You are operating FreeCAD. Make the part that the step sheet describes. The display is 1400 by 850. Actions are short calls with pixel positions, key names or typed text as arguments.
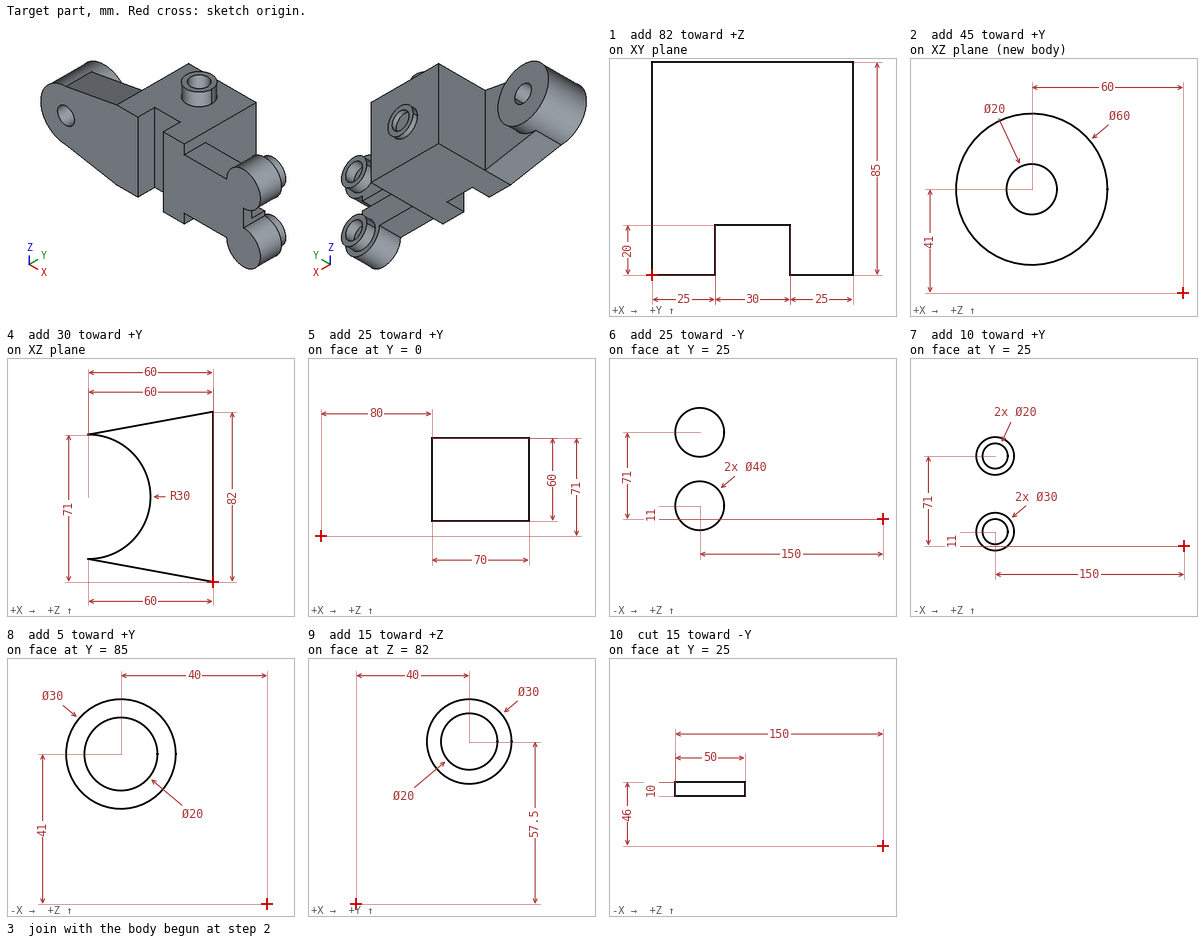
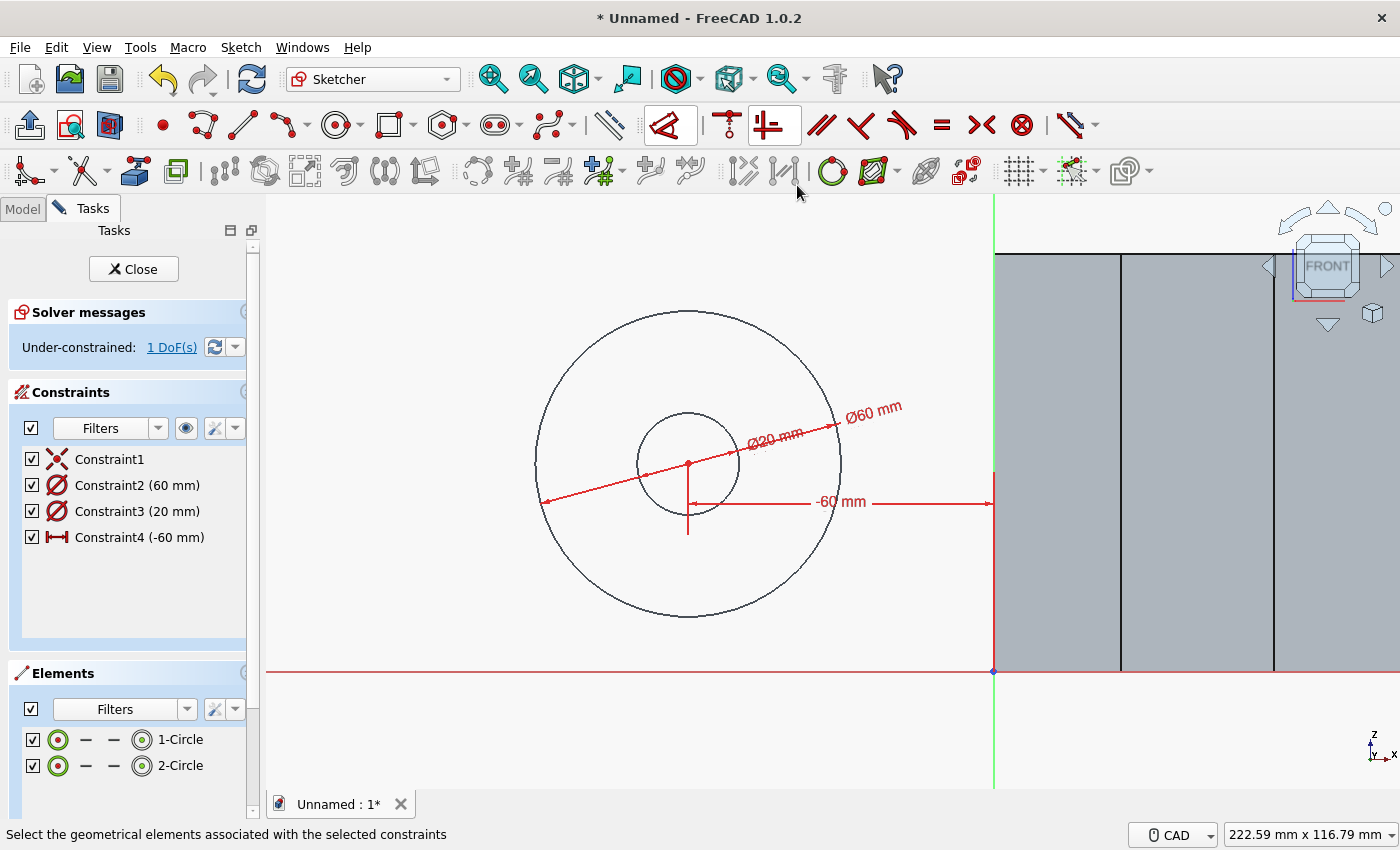
click(688, 464)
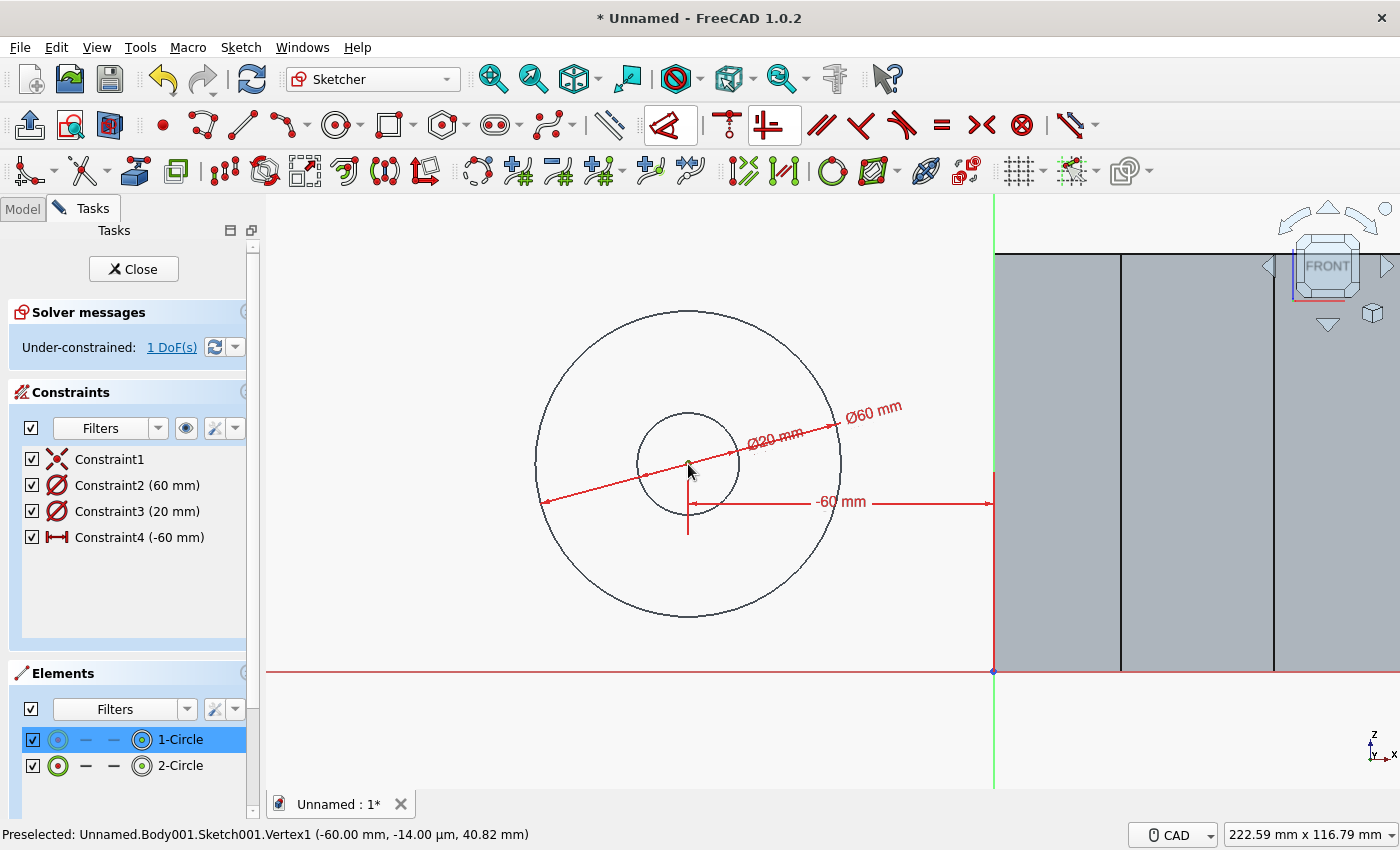
key(i)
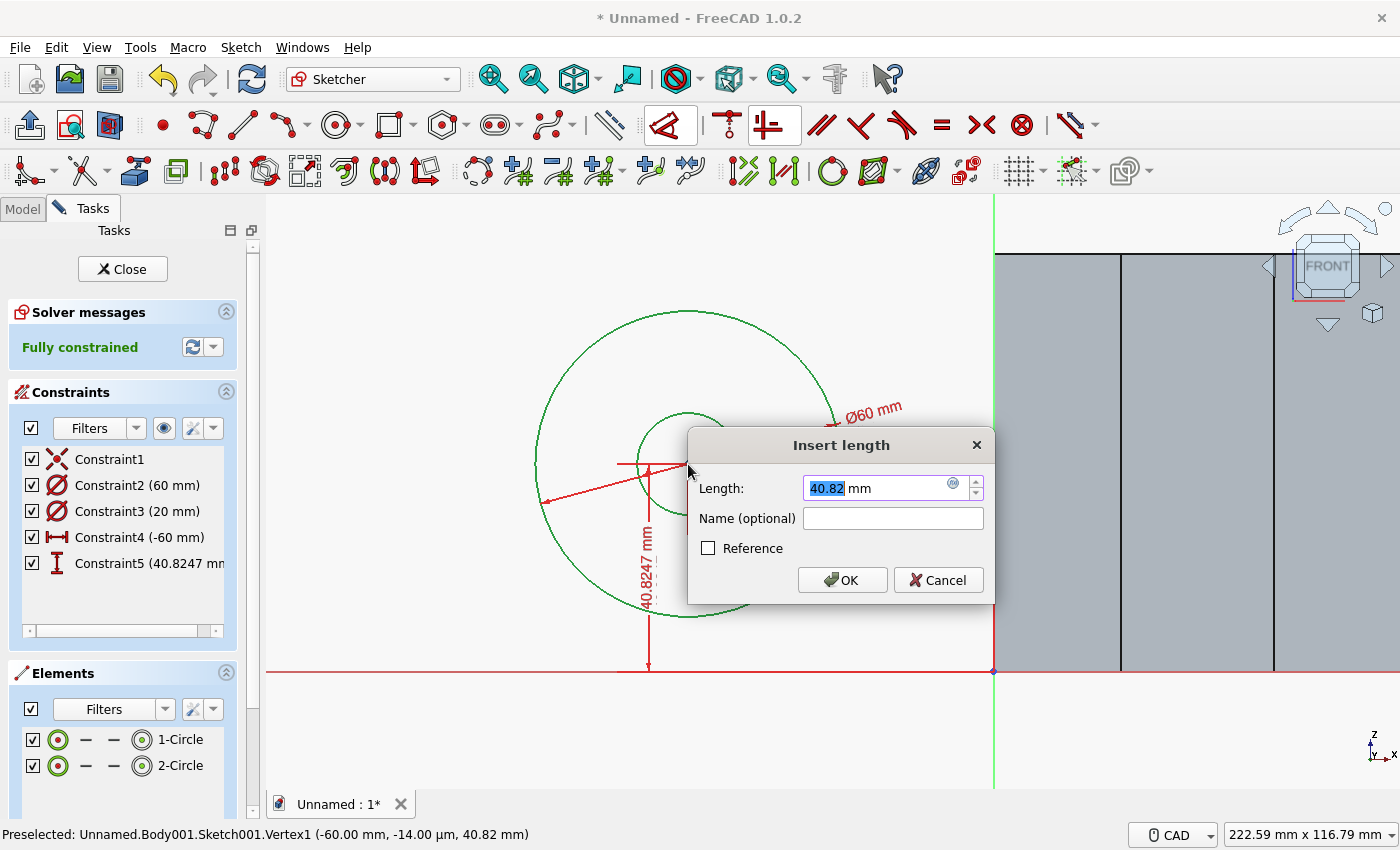
text(41)
key(Return)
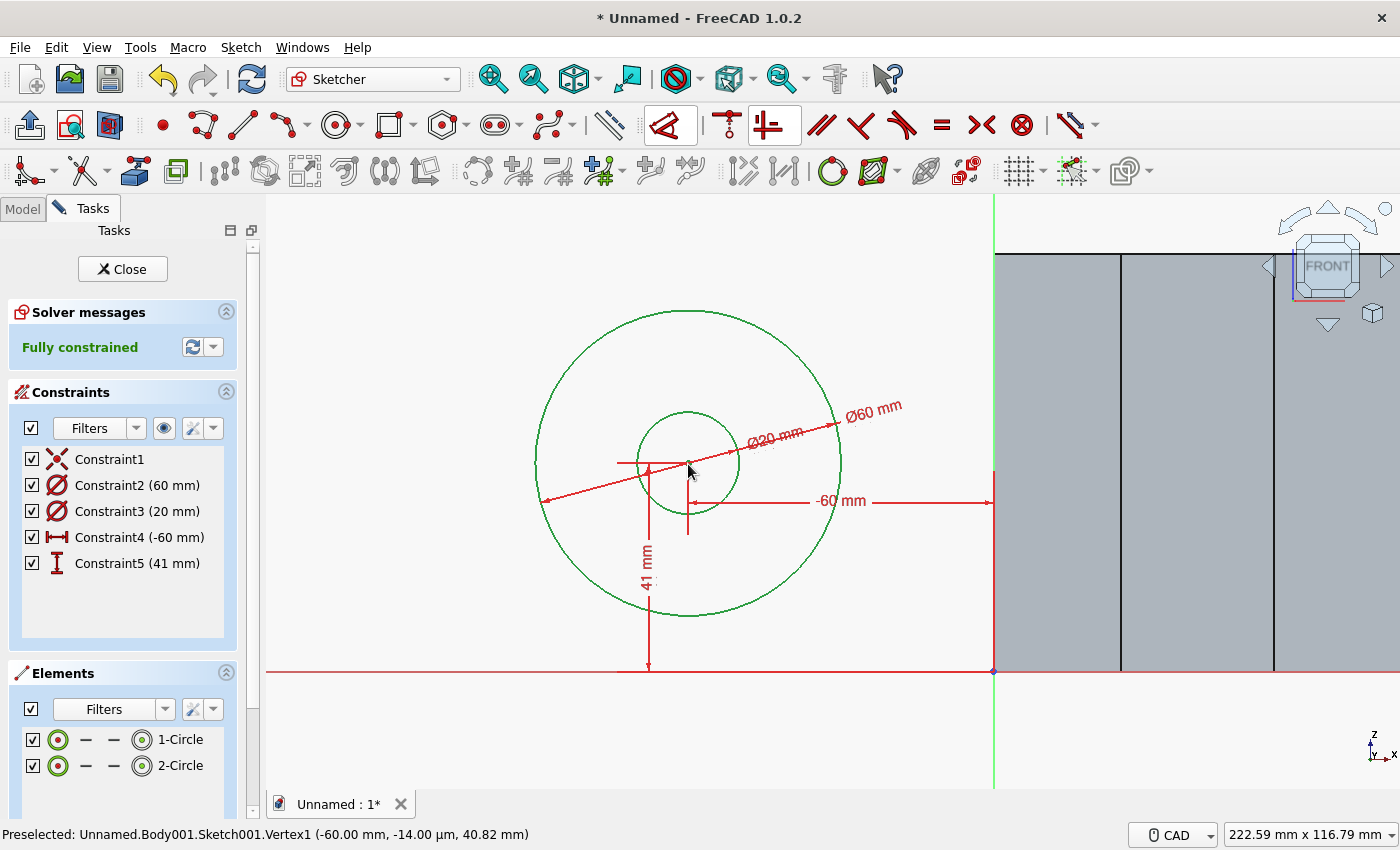
click(123, 269)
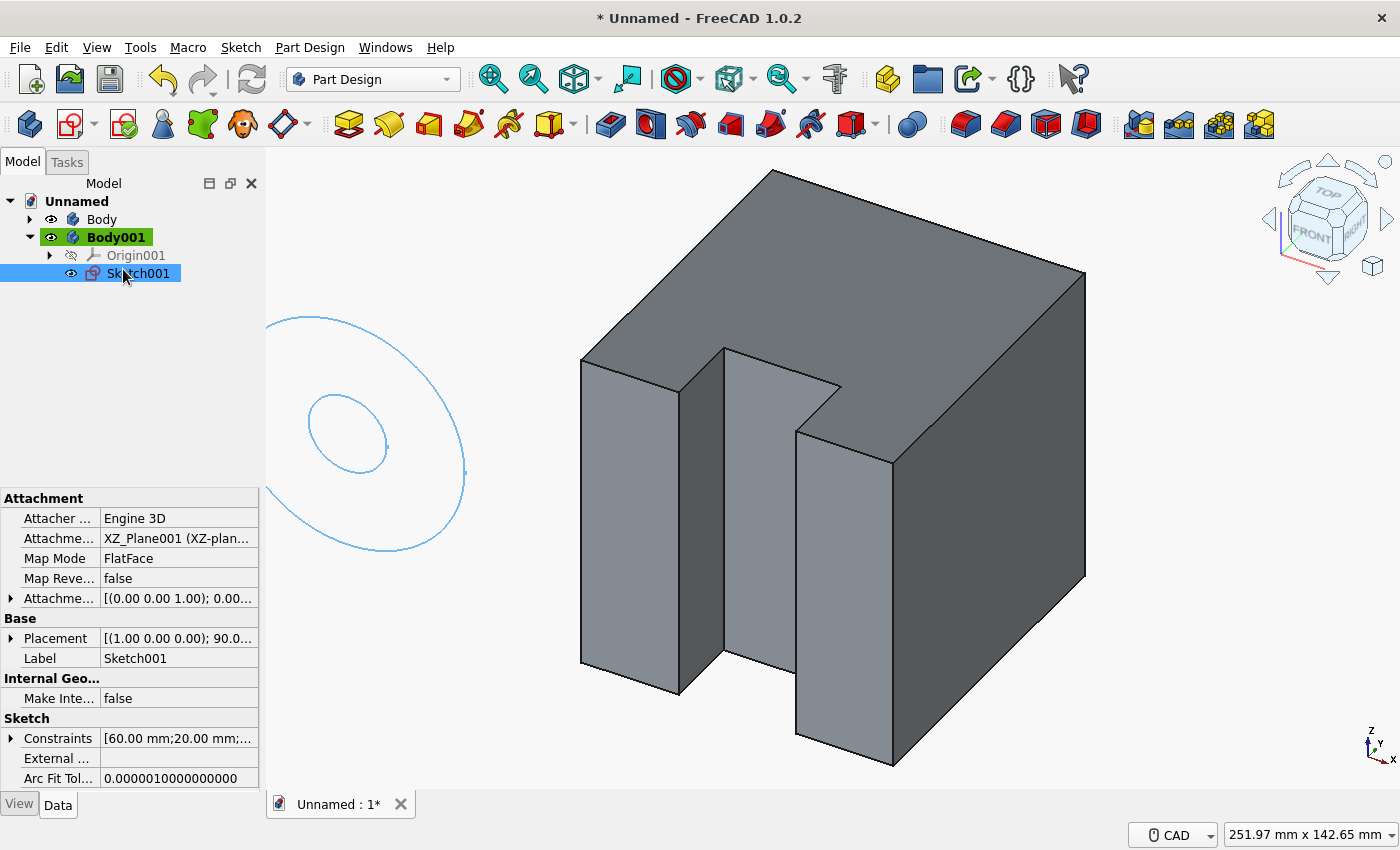
click(350, 124)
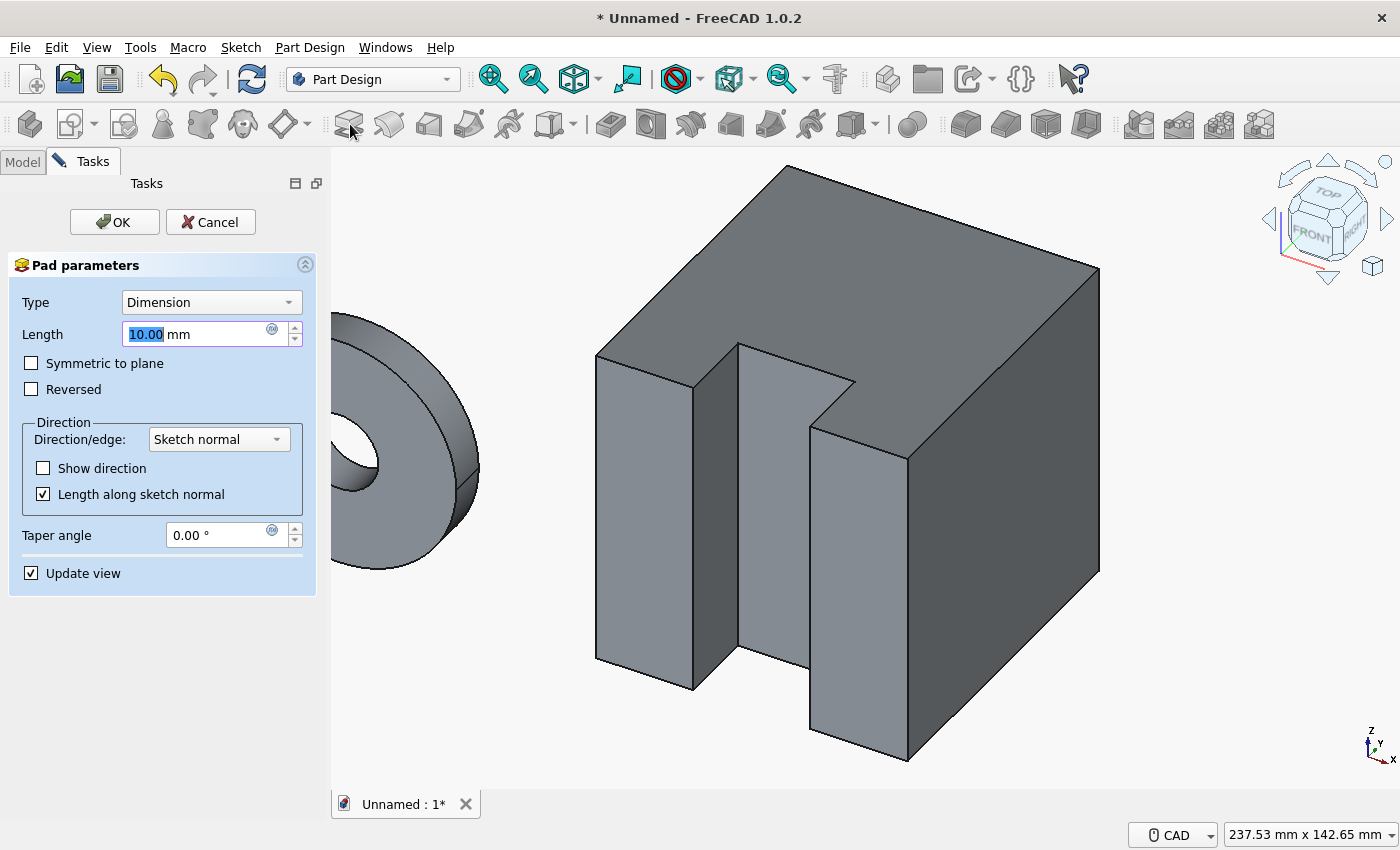
text(45)
key(Tab)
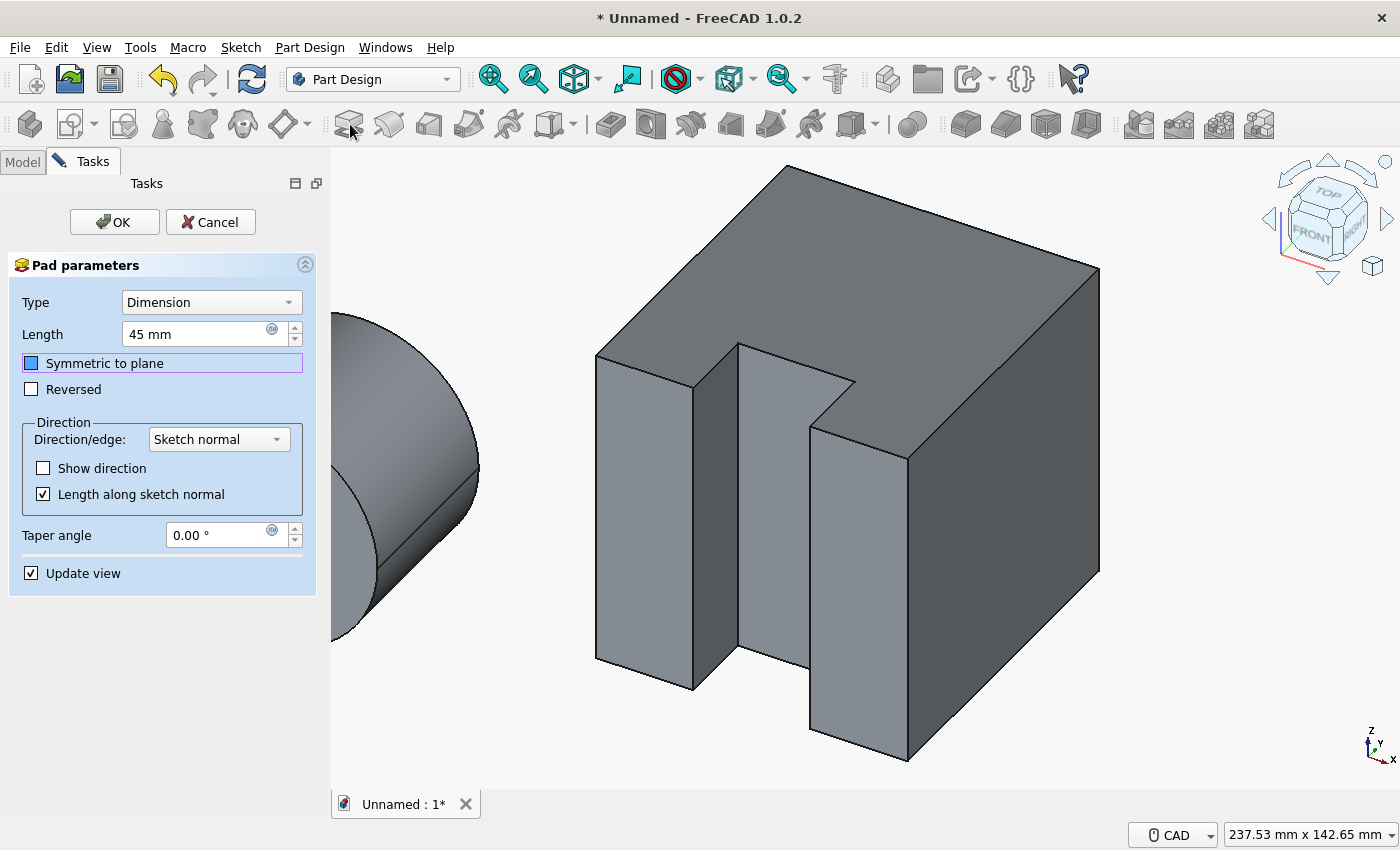
click(30, 389)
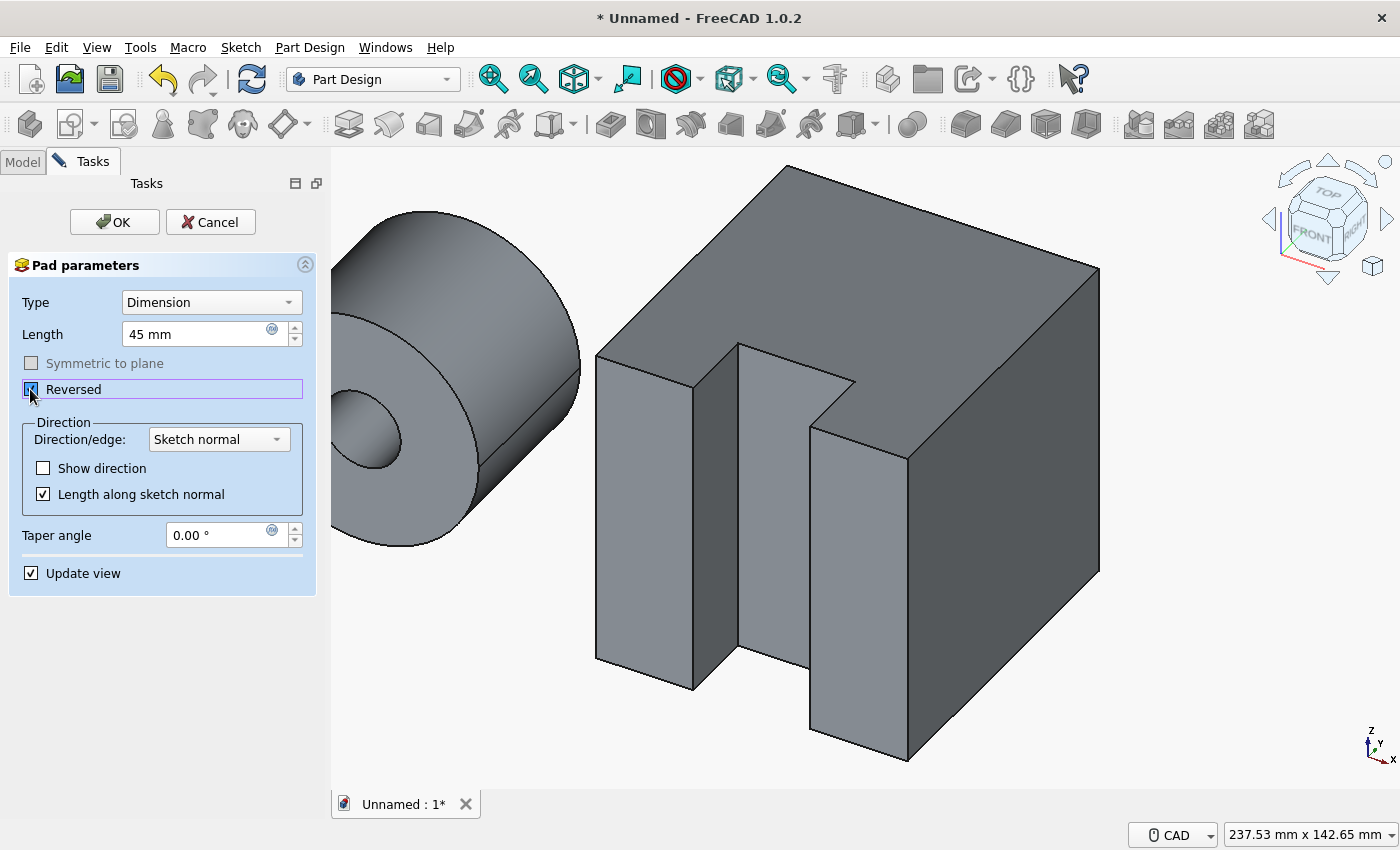
click(115, 222)